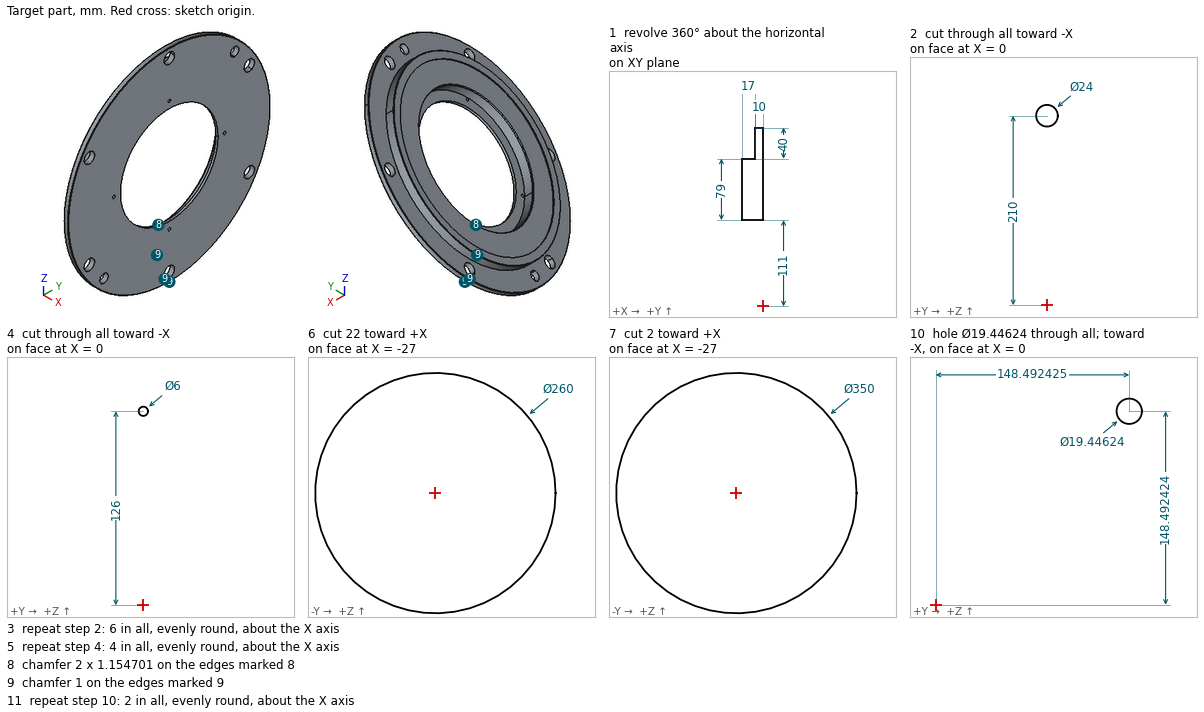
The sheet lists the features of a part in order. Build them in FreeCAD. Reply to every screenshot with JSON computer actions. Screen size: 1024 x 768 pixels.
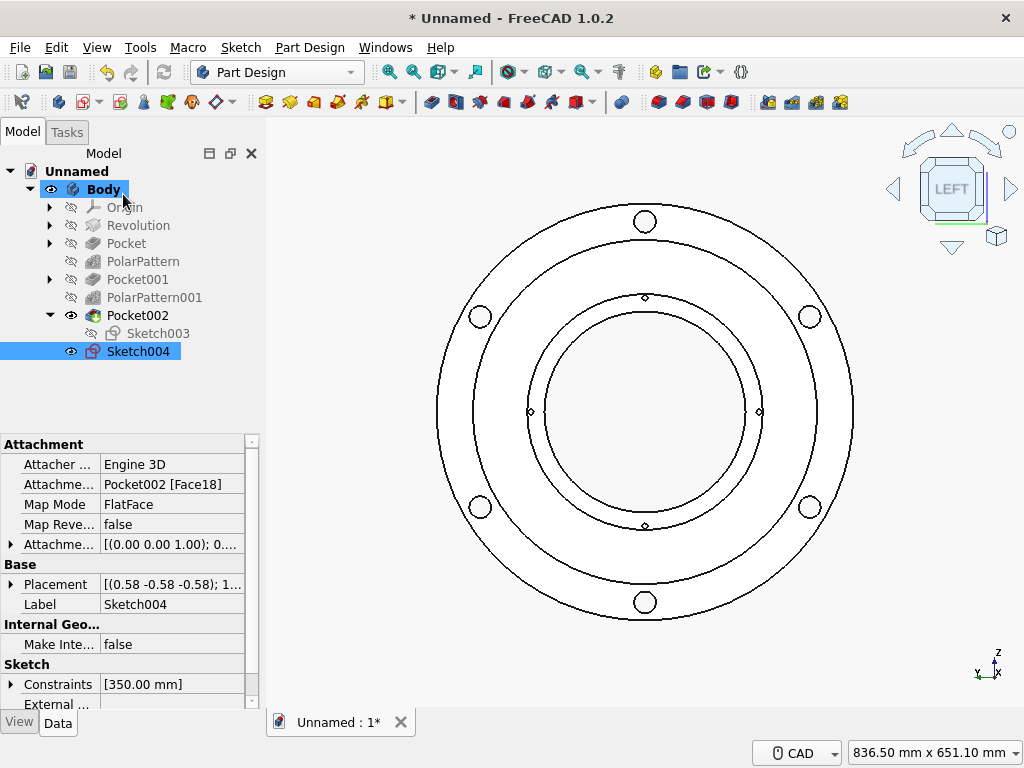
{"action": "left_click", "coordinate": [432, 102]}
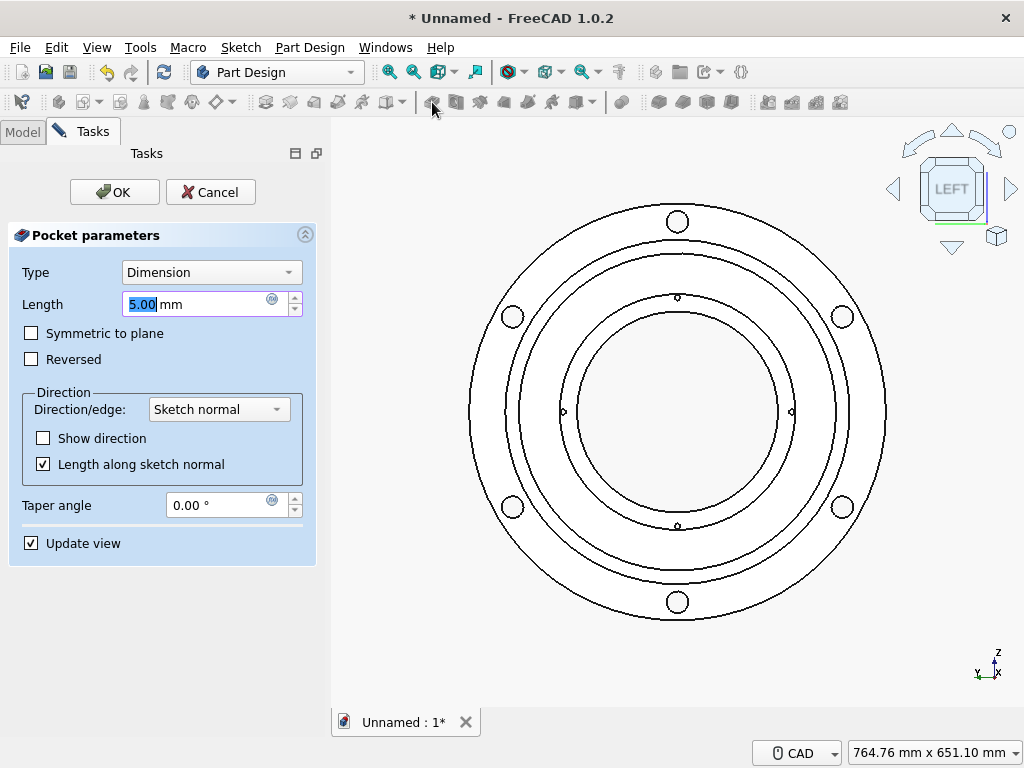
{"action": "type", "text": "2"}
{"action": "key", "text": "Tab"}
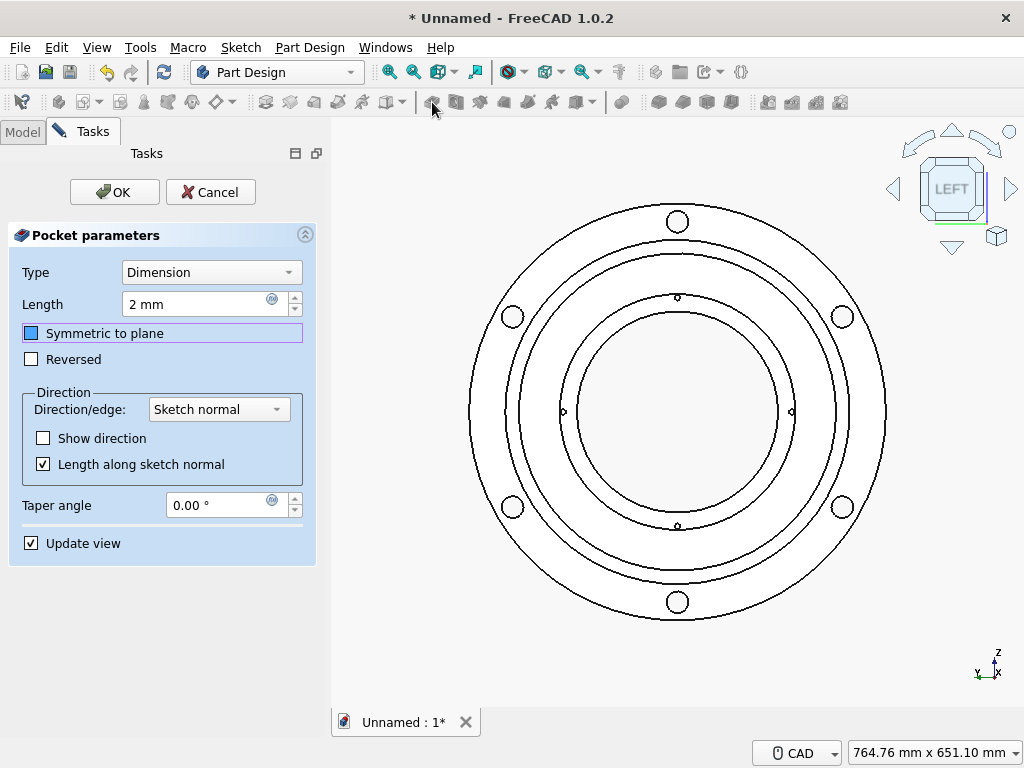
{"action": "left_click", "coordinate": [115, 192]}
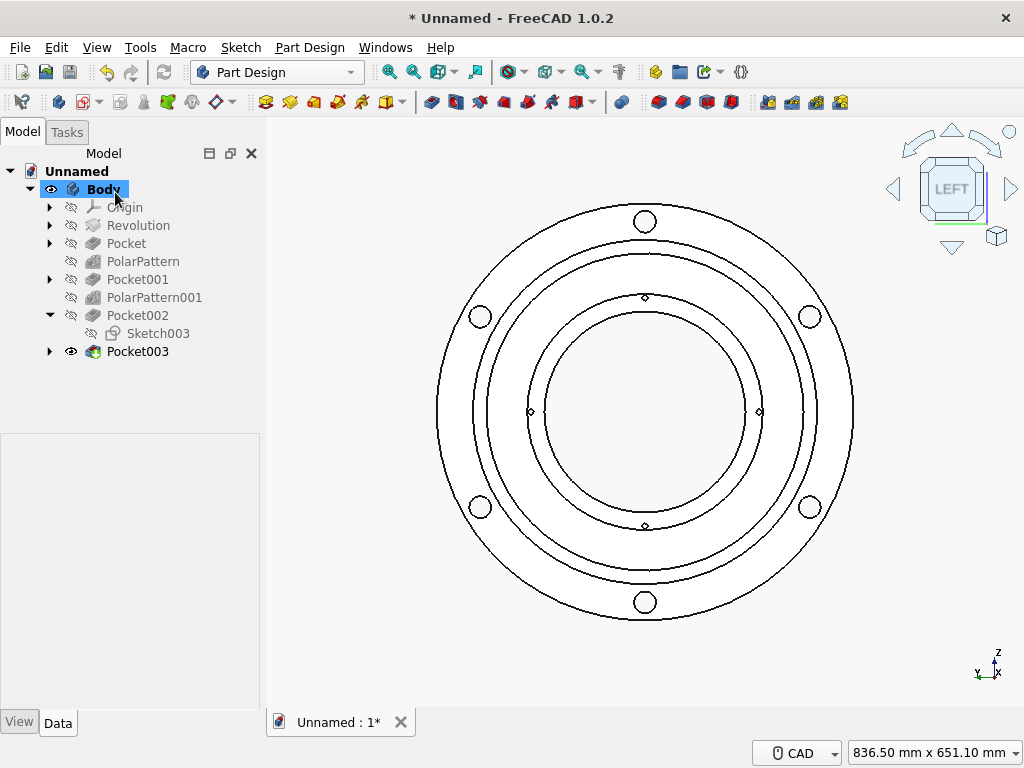
{"action": "left_click", "coordinate": [527, 411]}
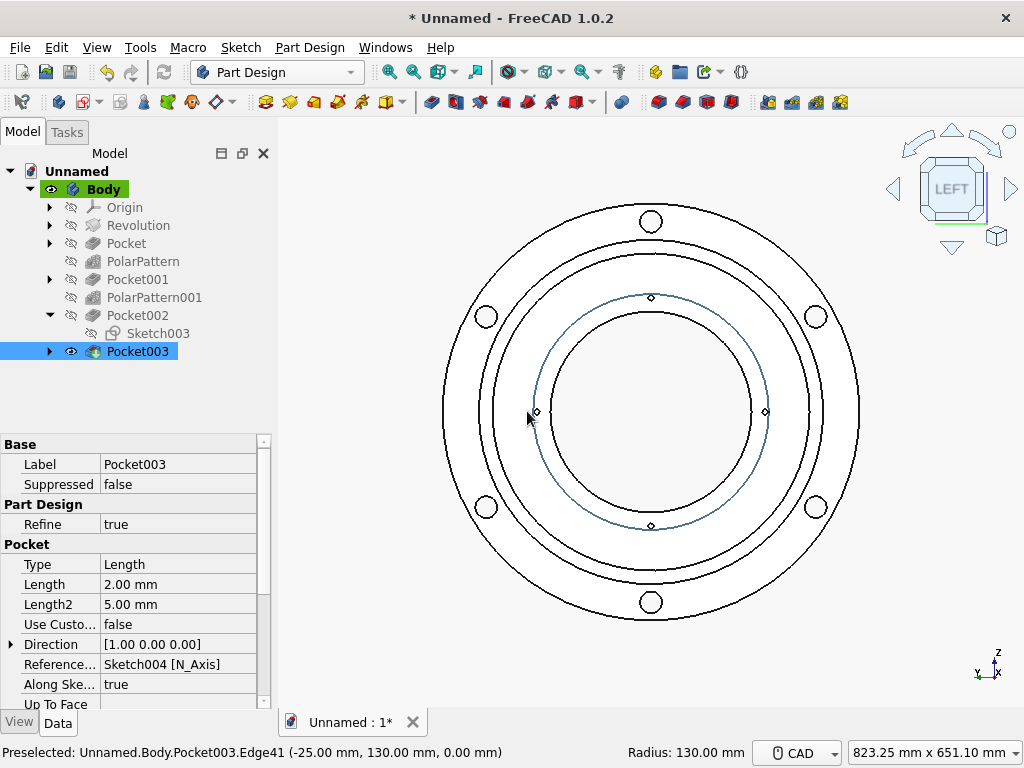
{"action": "left_click", "coordinate": [684, 102]}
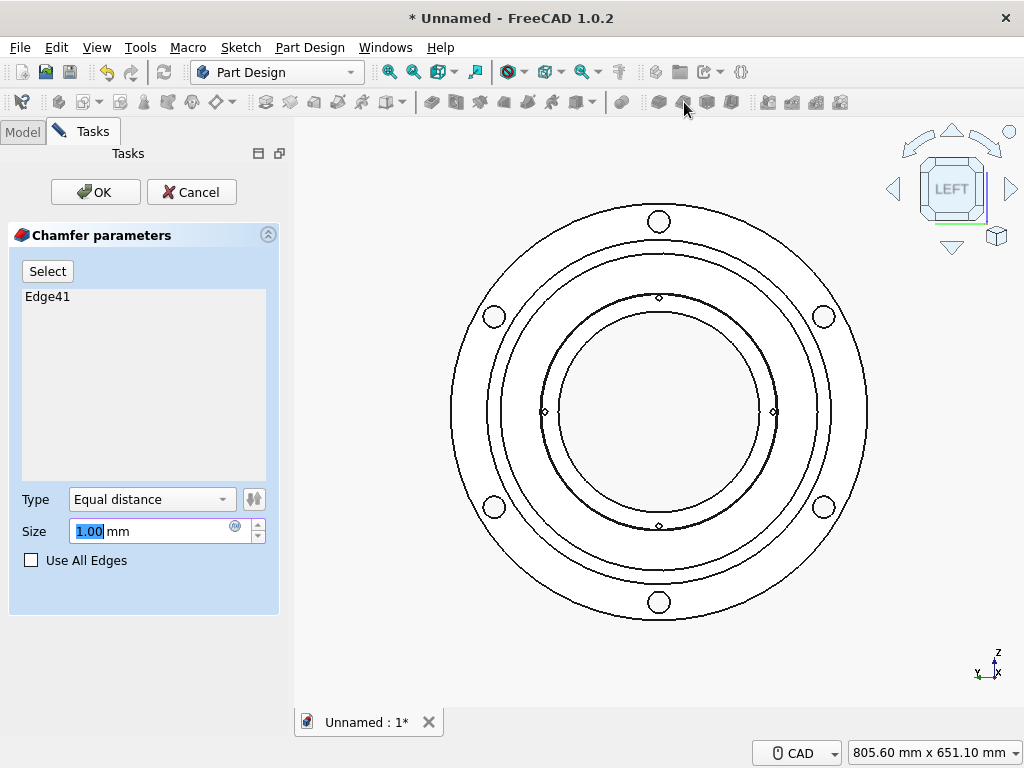
{"action": "type", "text": "2"}
{"action": "key", "text": "Tab"}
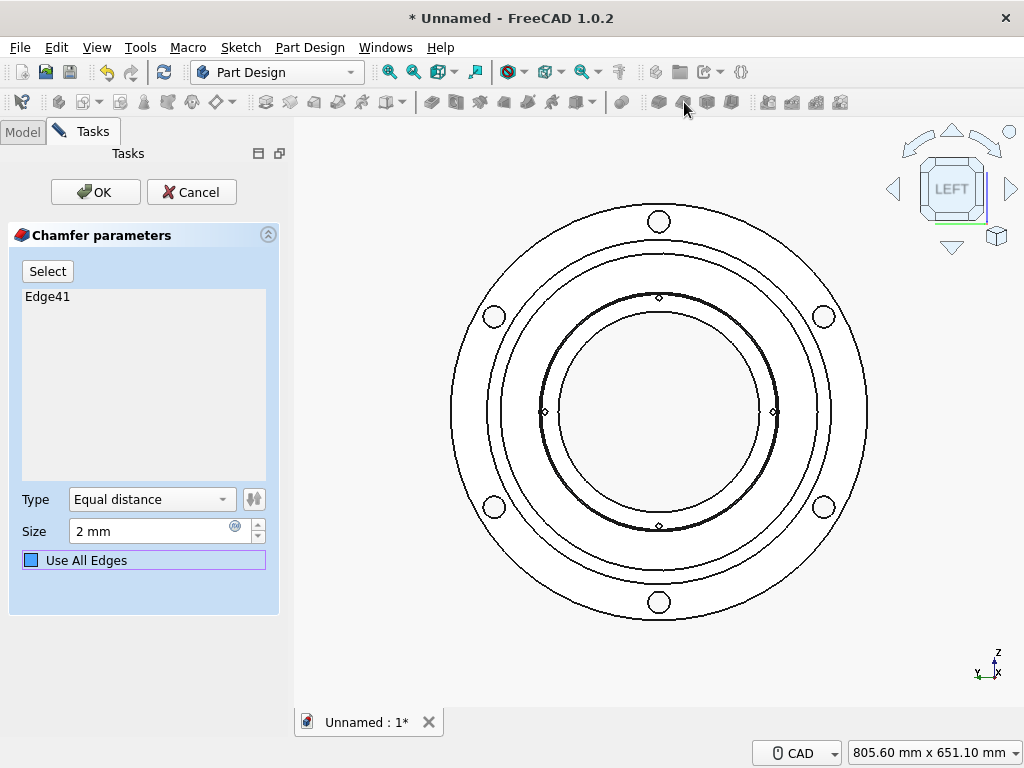
{"action": "left_click", "coordinate": [153, 500]}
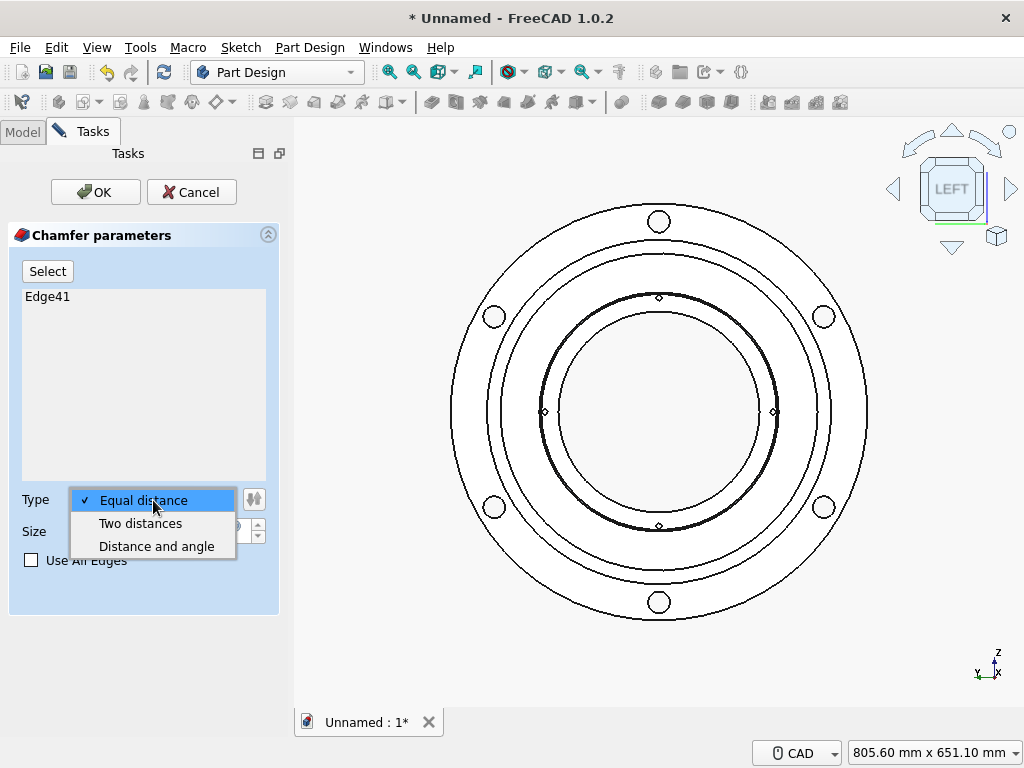
{"action": "left_click", "coordinate": [152, 524]}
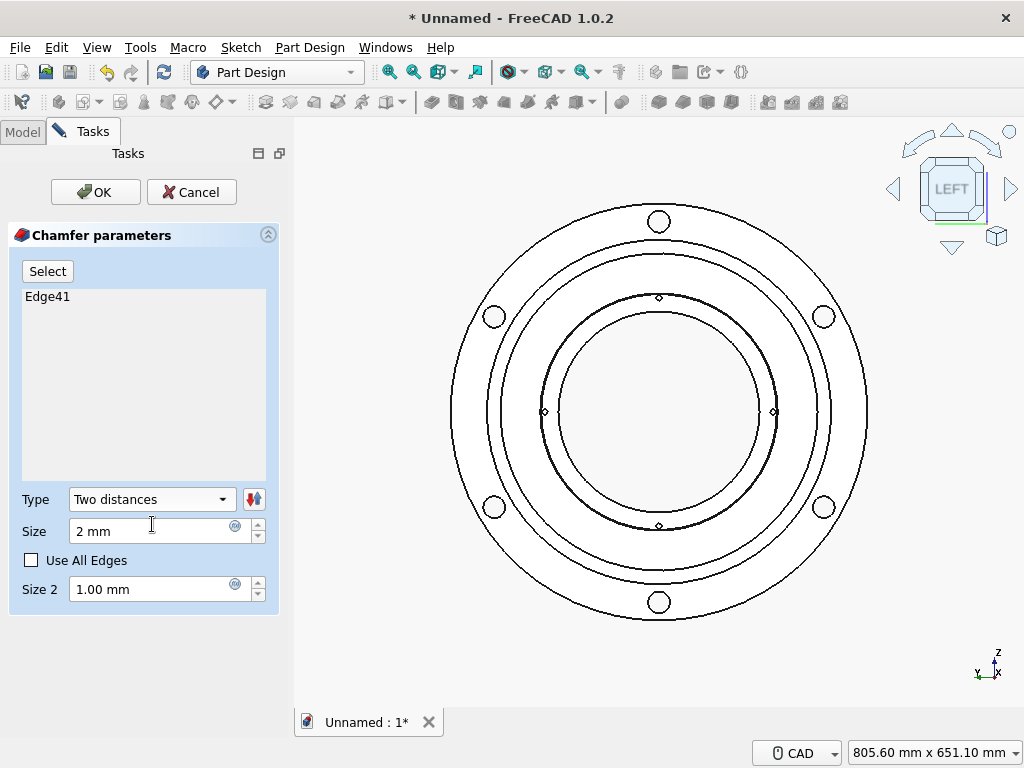
{"action": "triple_click", "coordinate": [160, 589]}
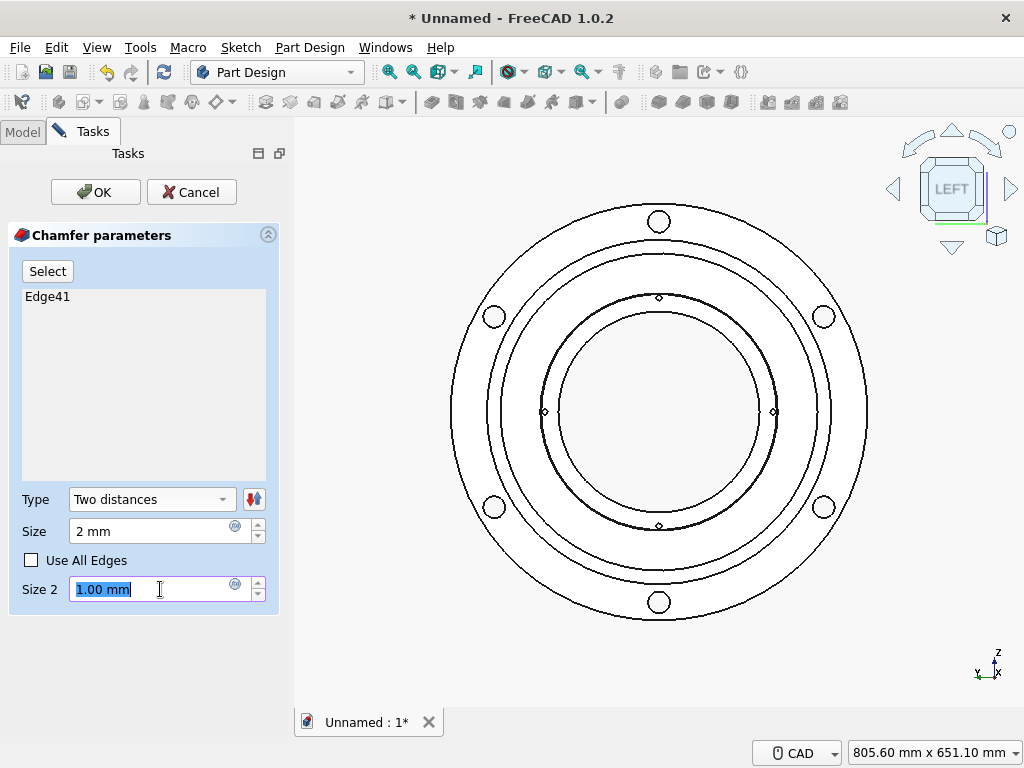
{"action": "type", "text": "1.154701"}
{"action": "key", "text": "Tab"}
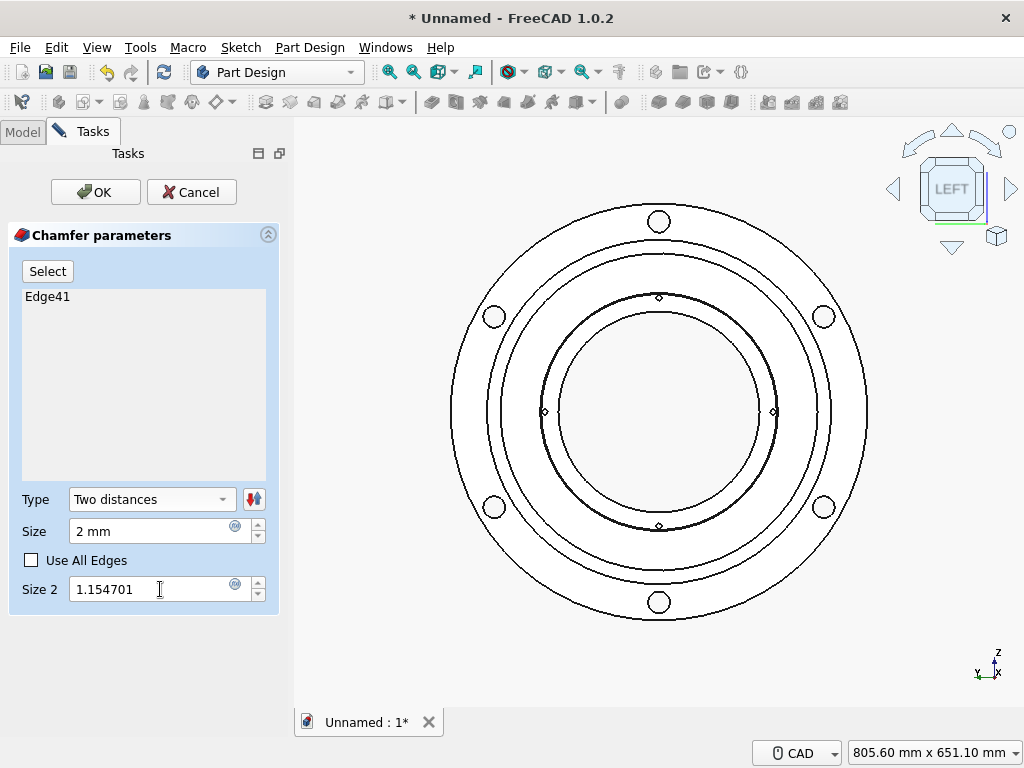
{"action": "left_click", "coordinate": [96, 192]}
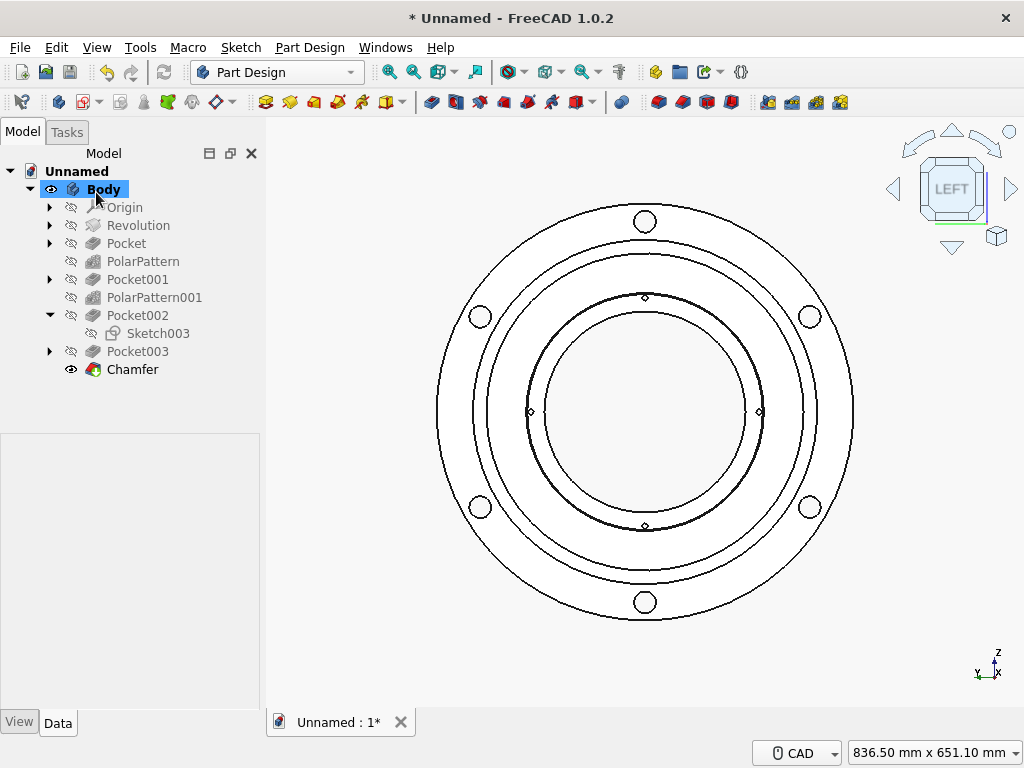
{"action": "left_click", "coordinate": [817, 411]}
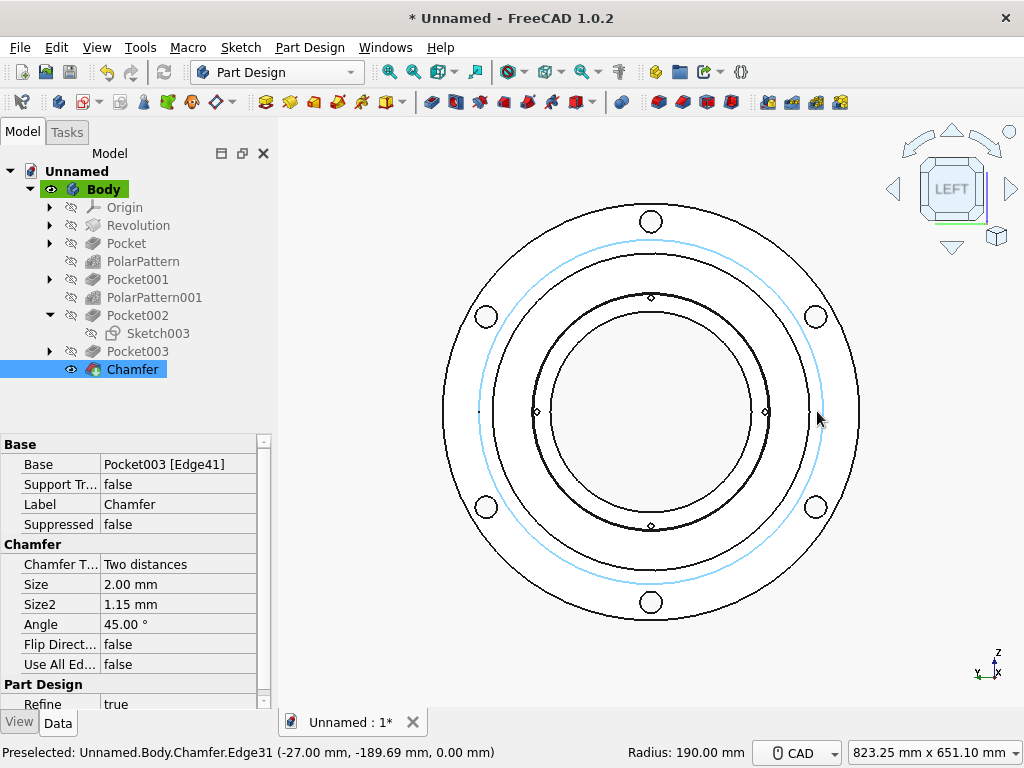
{"action": "left_click", "coordinate": [859, 411], "text": "ctrl"}